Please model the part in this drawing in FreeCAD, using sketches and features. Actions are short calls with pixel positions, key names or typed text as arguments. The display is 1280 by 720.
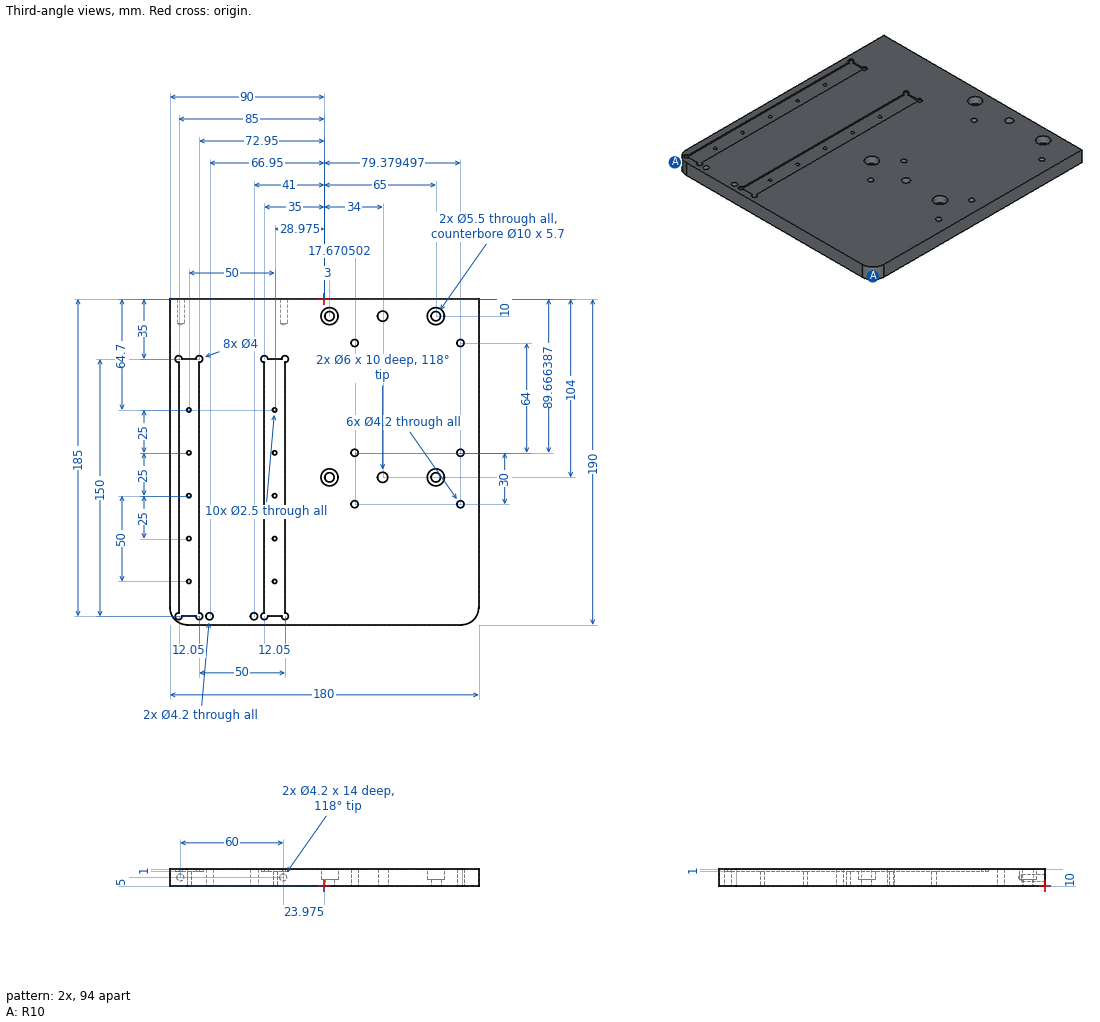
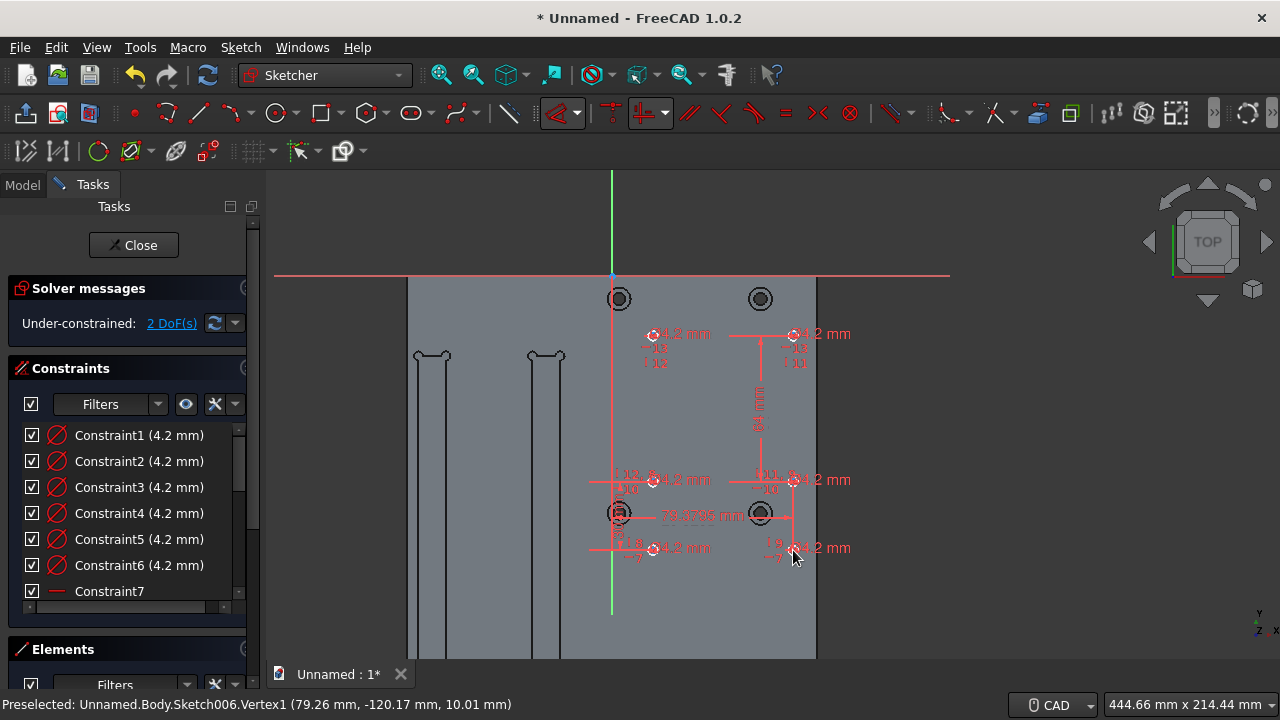
click(653, 550)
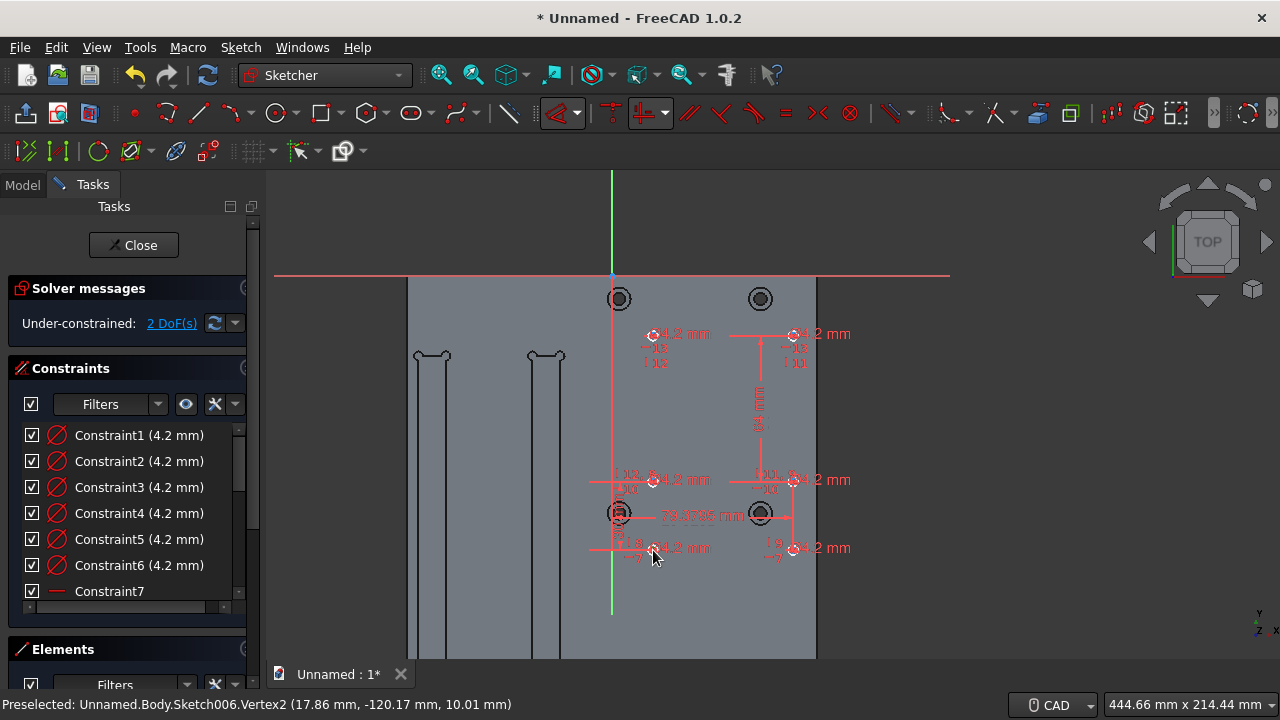
key(l)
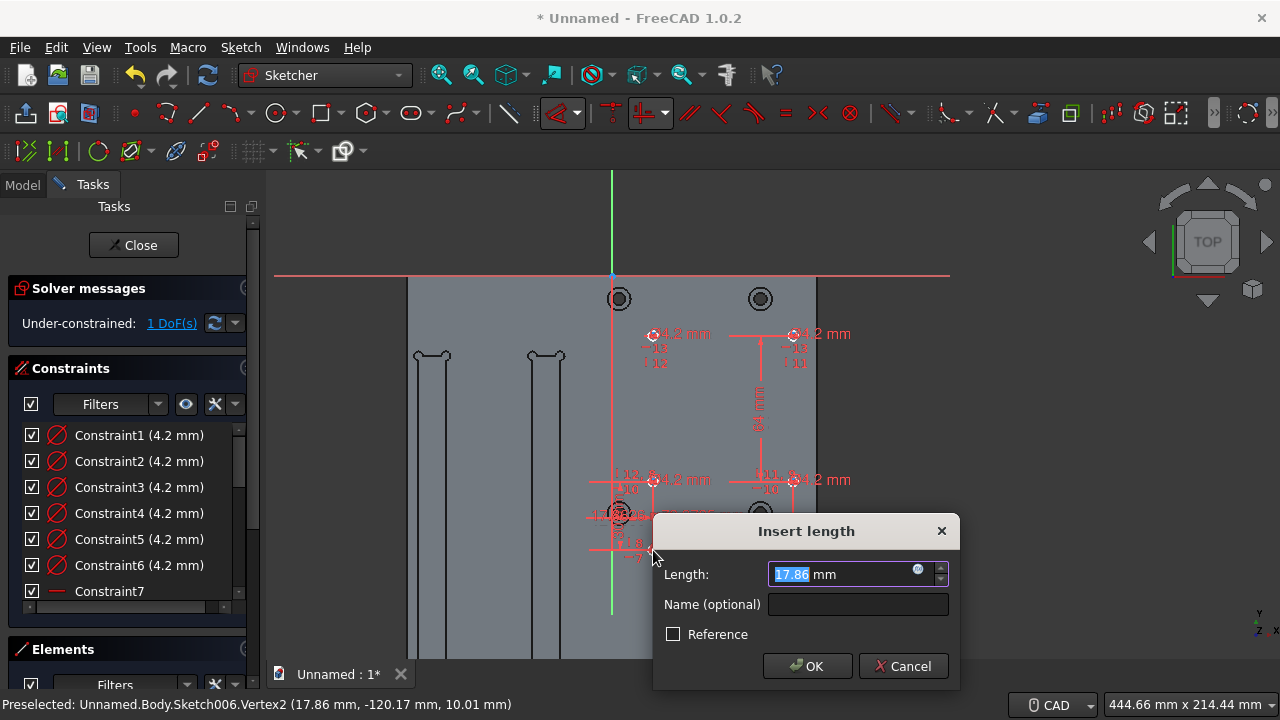
text(17.670502)
key(Return)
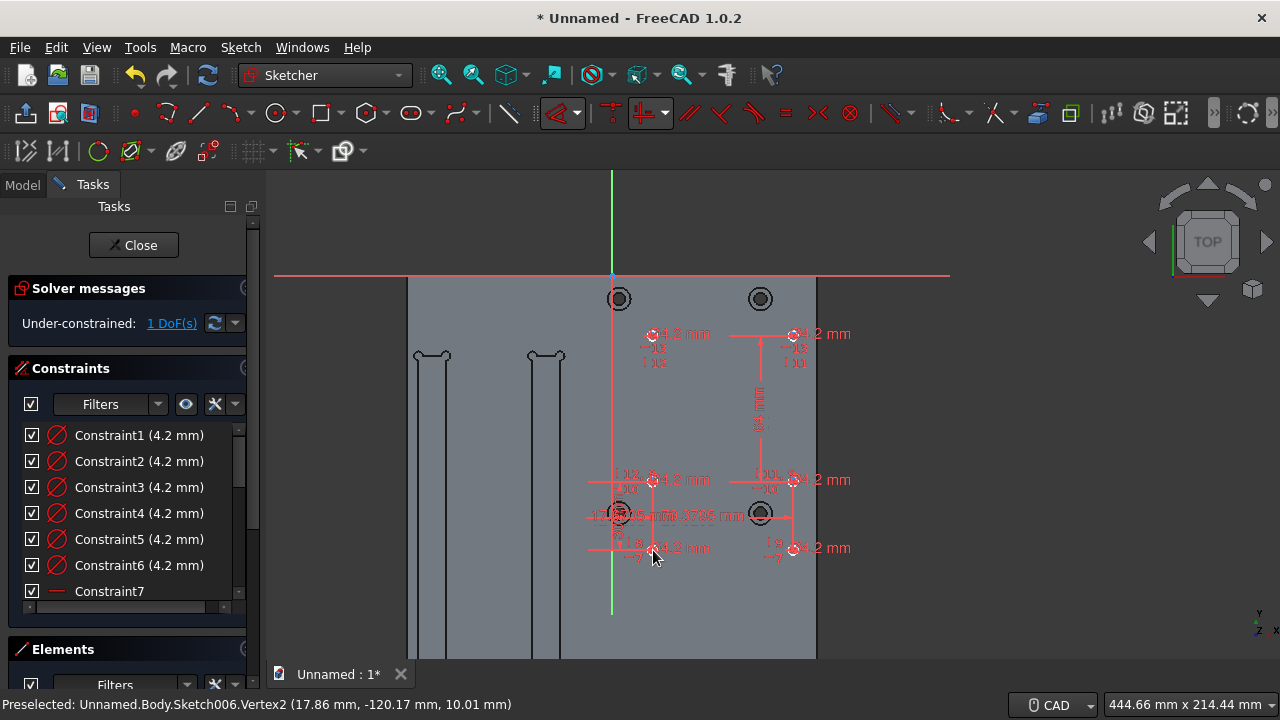
click(653, 482)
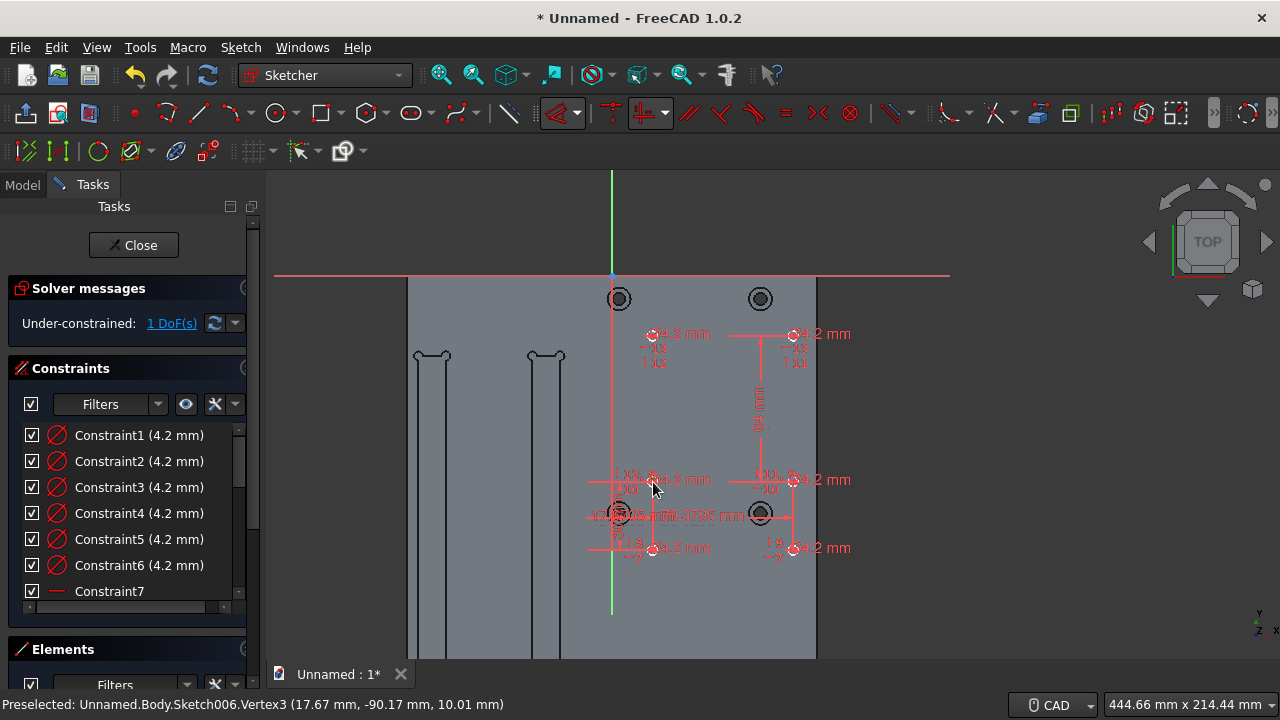
click(580, 114)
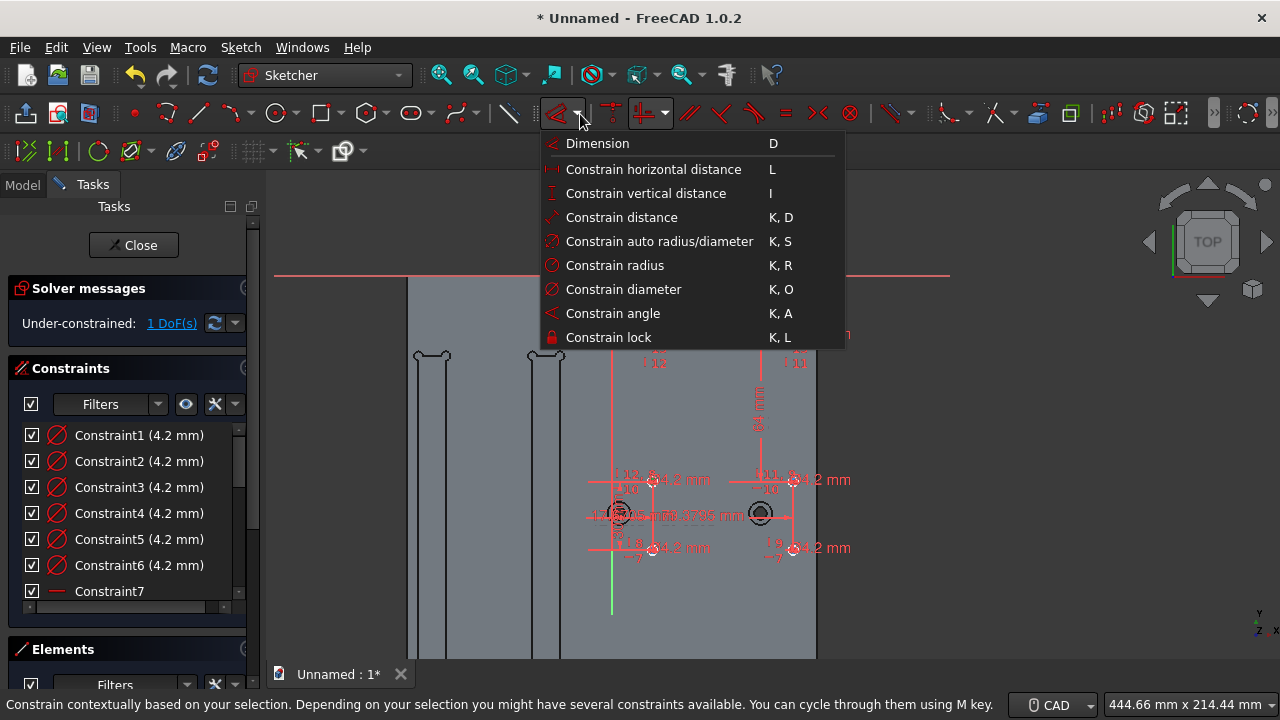
click(693, 193)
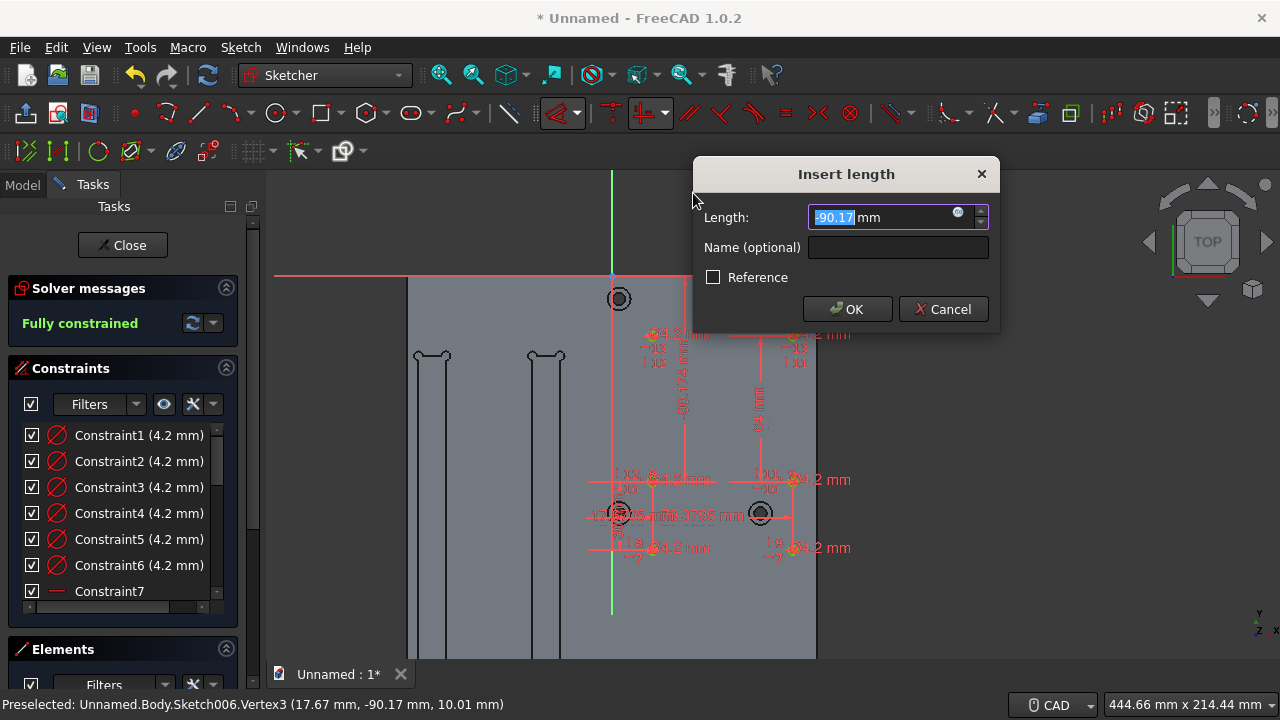
text(-89.666387)
key(Return)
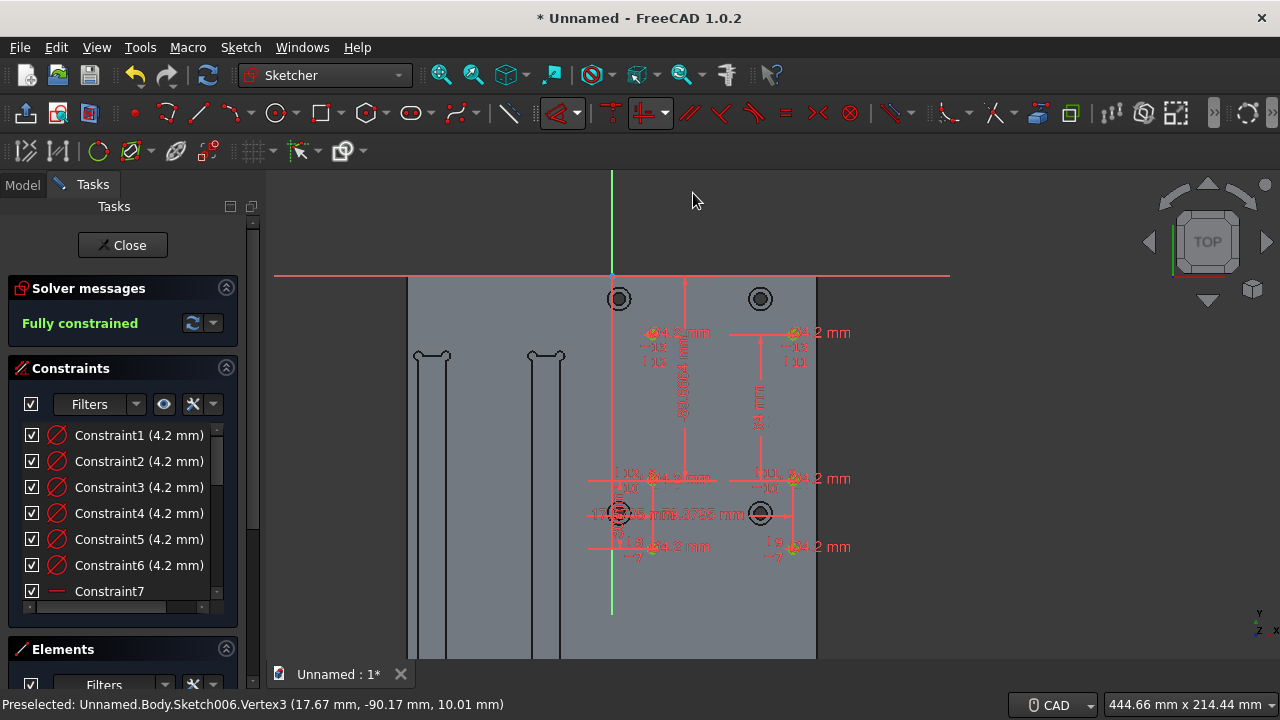
click(123, 245)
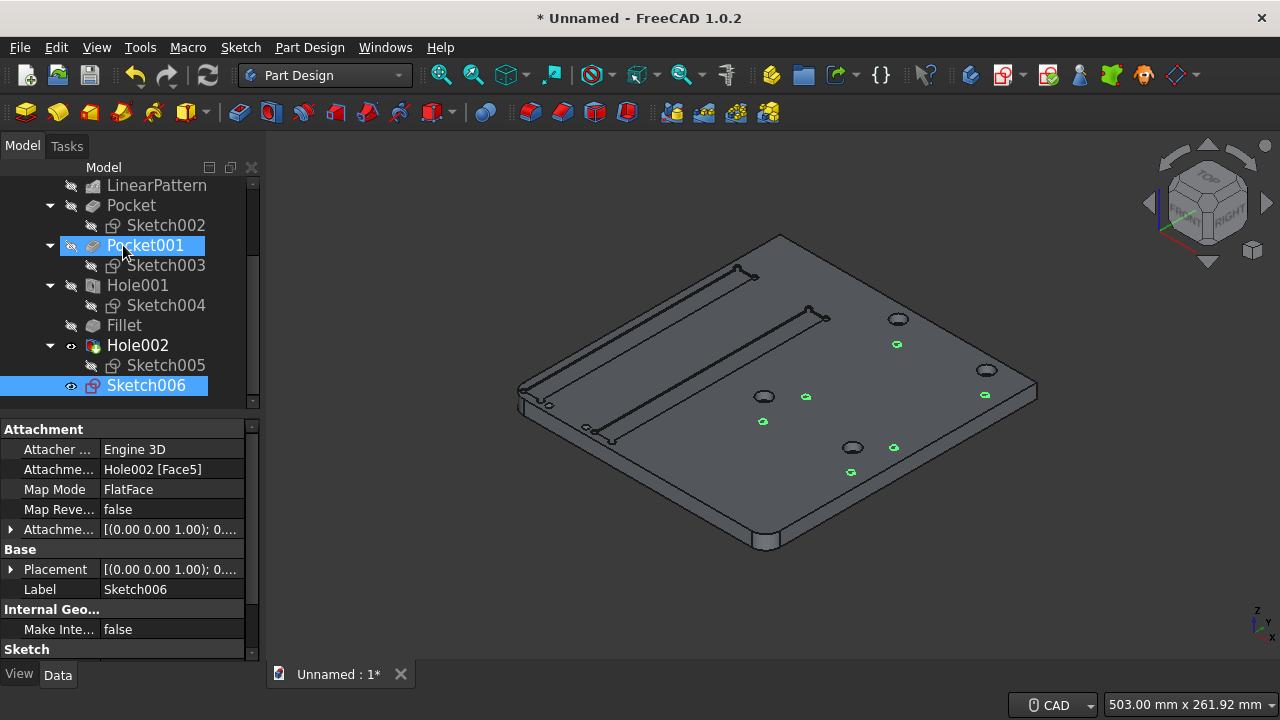
click(272, 112)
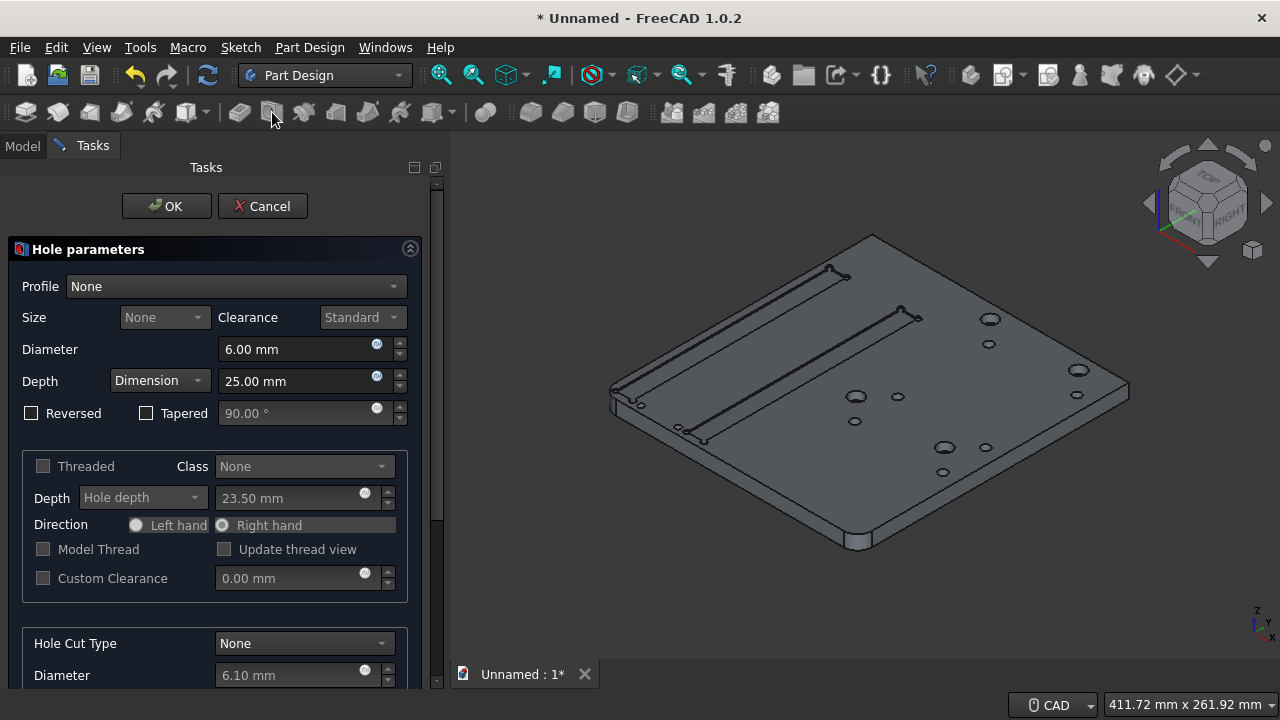
triple_click(305, 349)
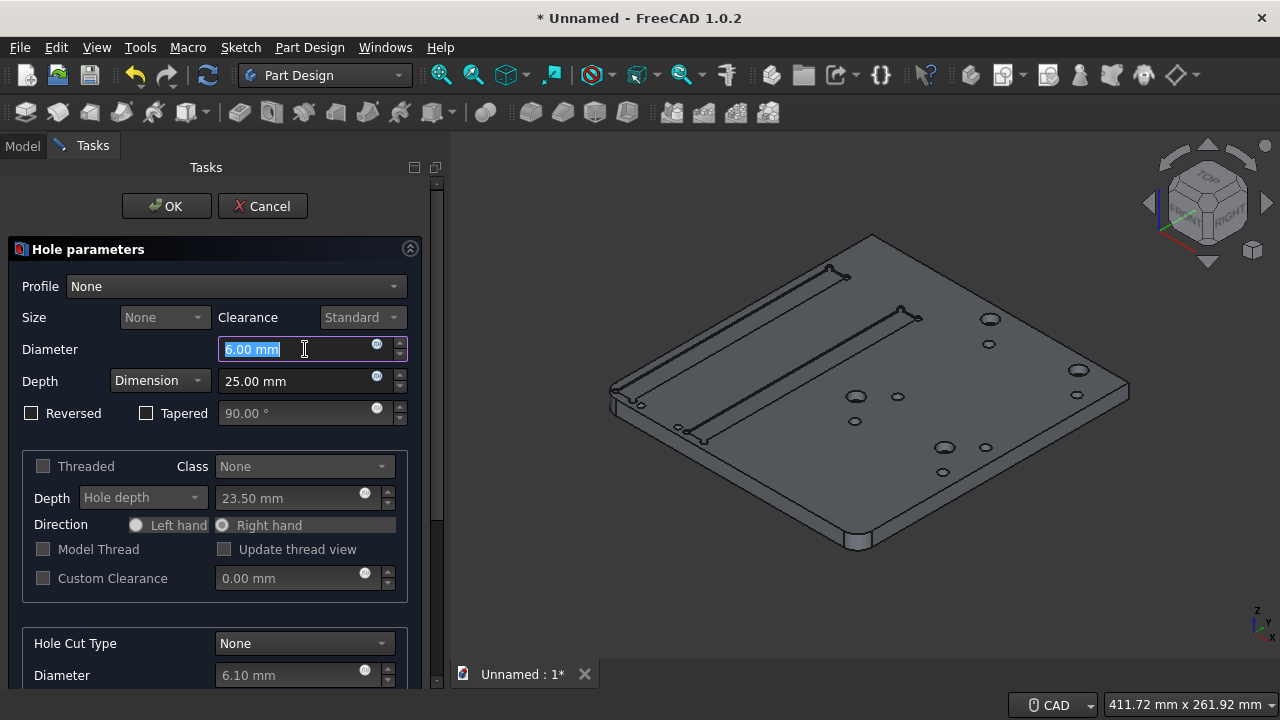
text(4.2)
key(Tab)